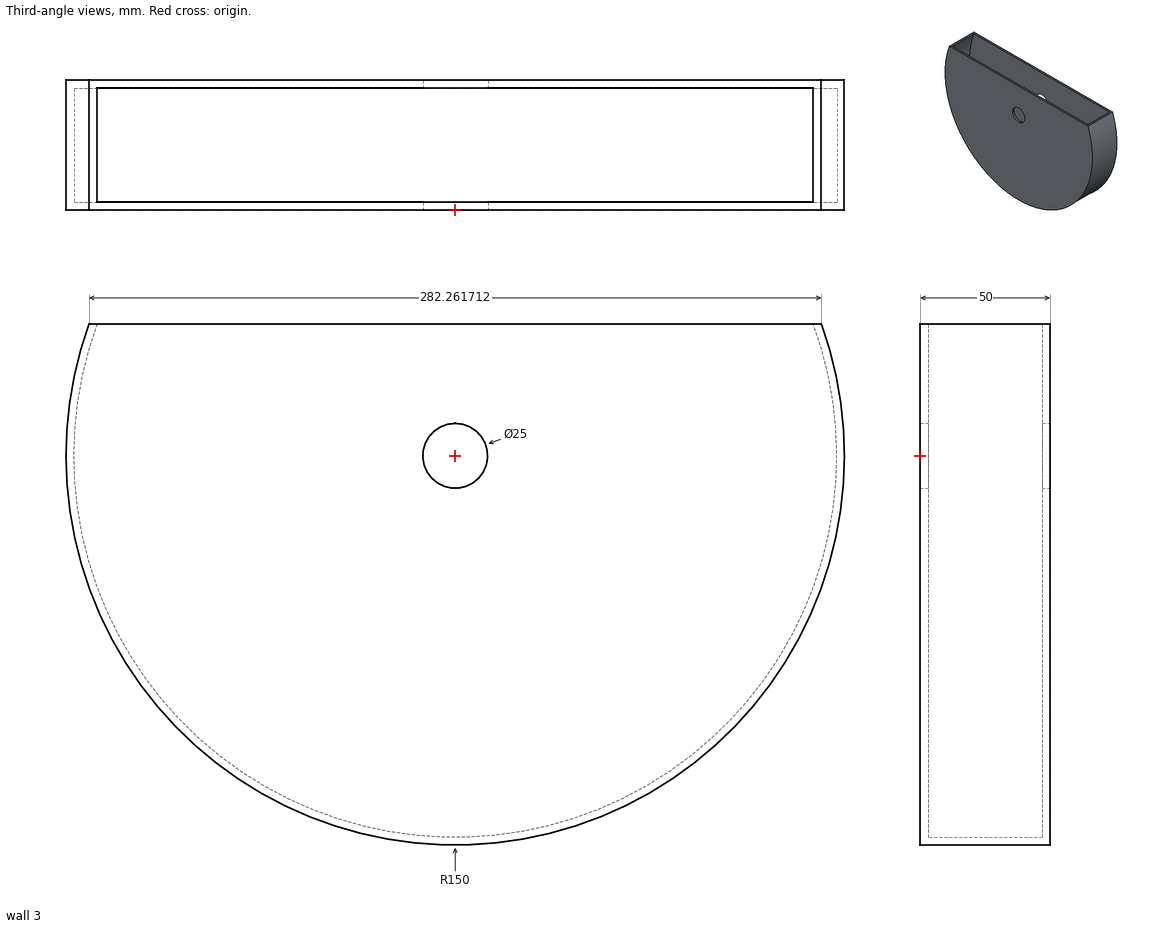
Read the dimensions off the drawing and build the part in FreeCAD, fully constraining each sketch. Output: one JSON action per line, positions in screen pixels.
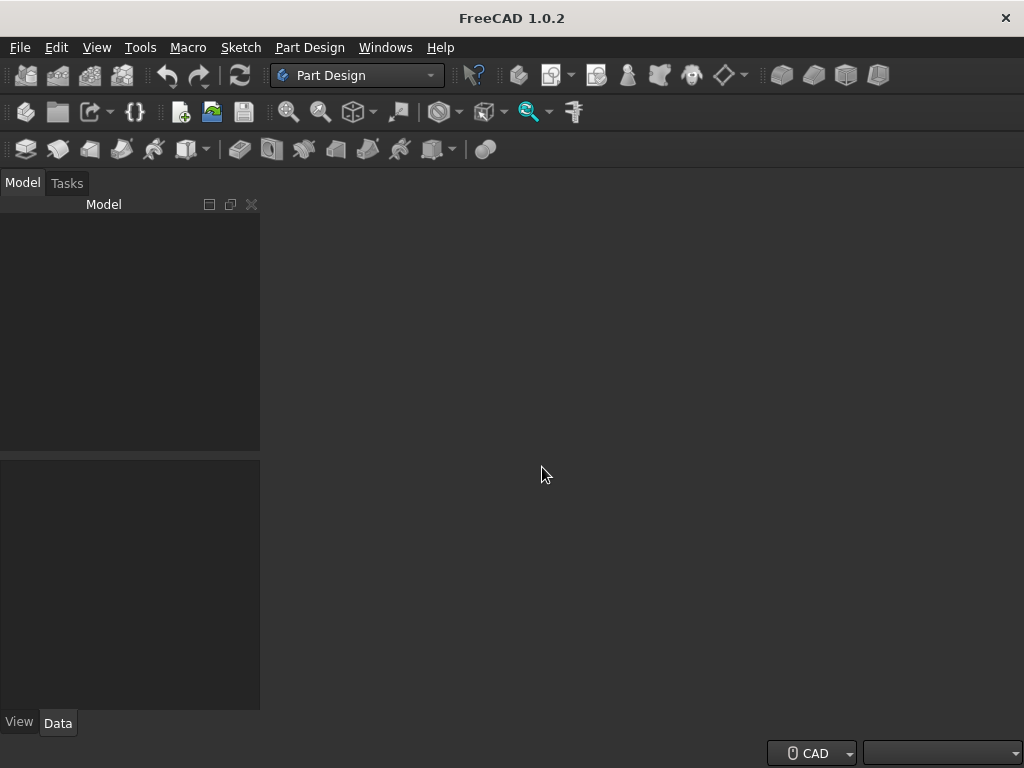
{"action": "key", "text": "ctrl+n"}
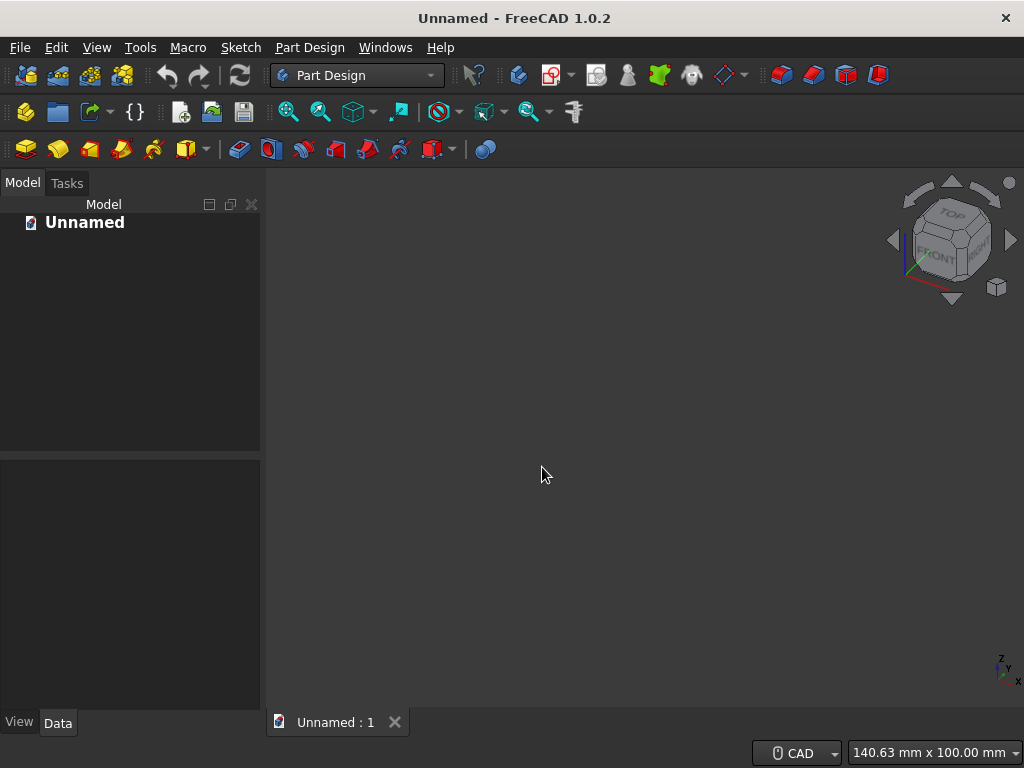
{"action": "left_click", "coordinate": [552, 76]}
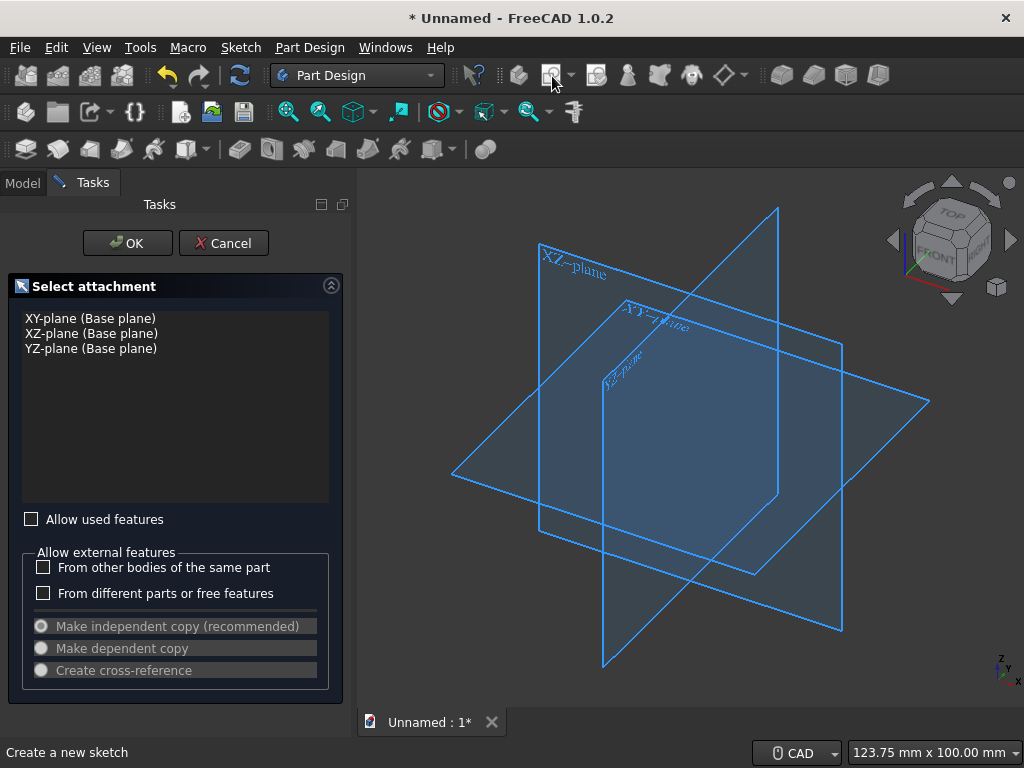
{"action": "left_click", "coordinate": [82, 334]}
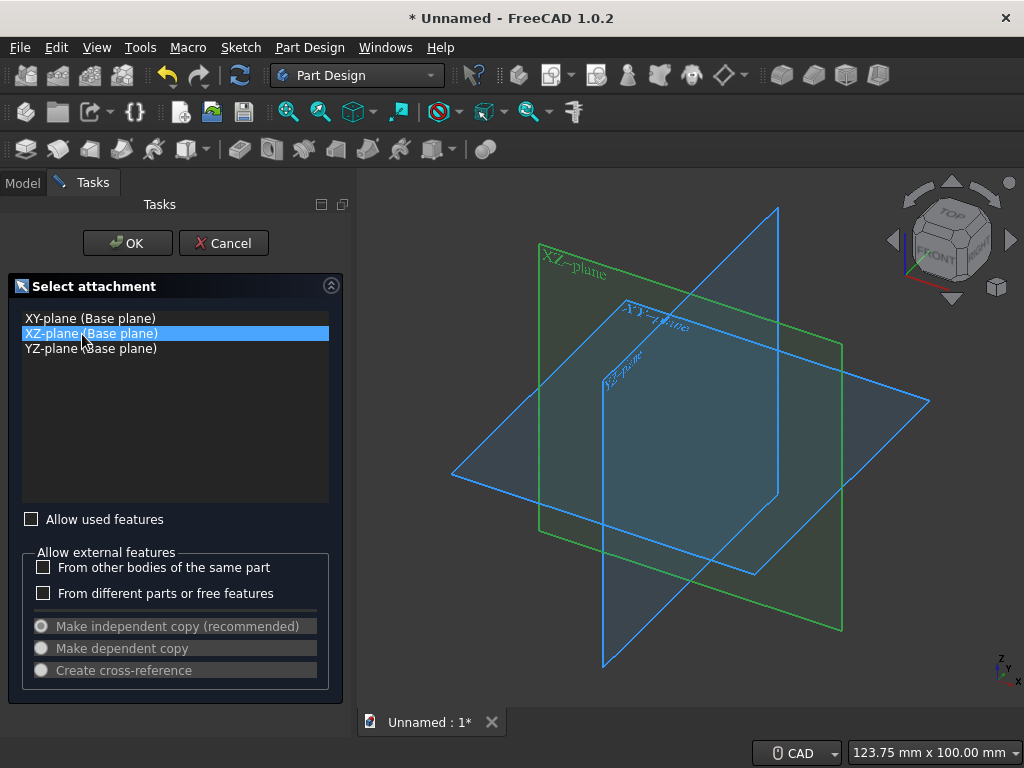
{"action": "left_click", "coordinate": [128, 243]}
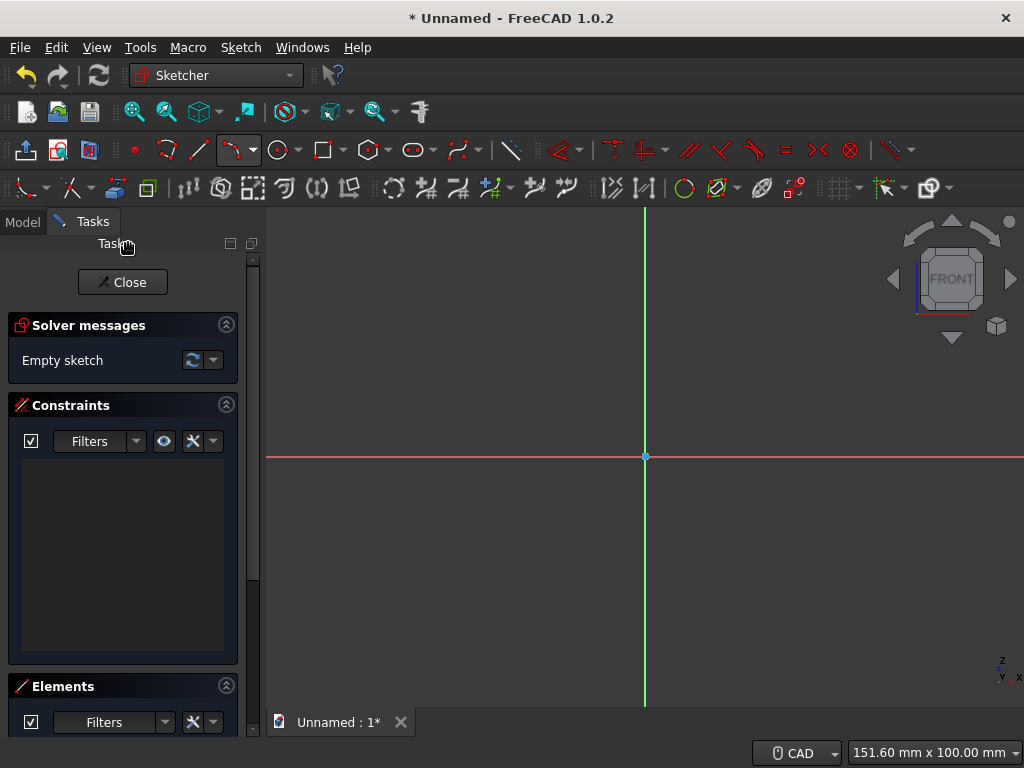
{"action": "scroll", "coordinate": [547, 350], "scroll_direction": "down", "scroll_amount": 6}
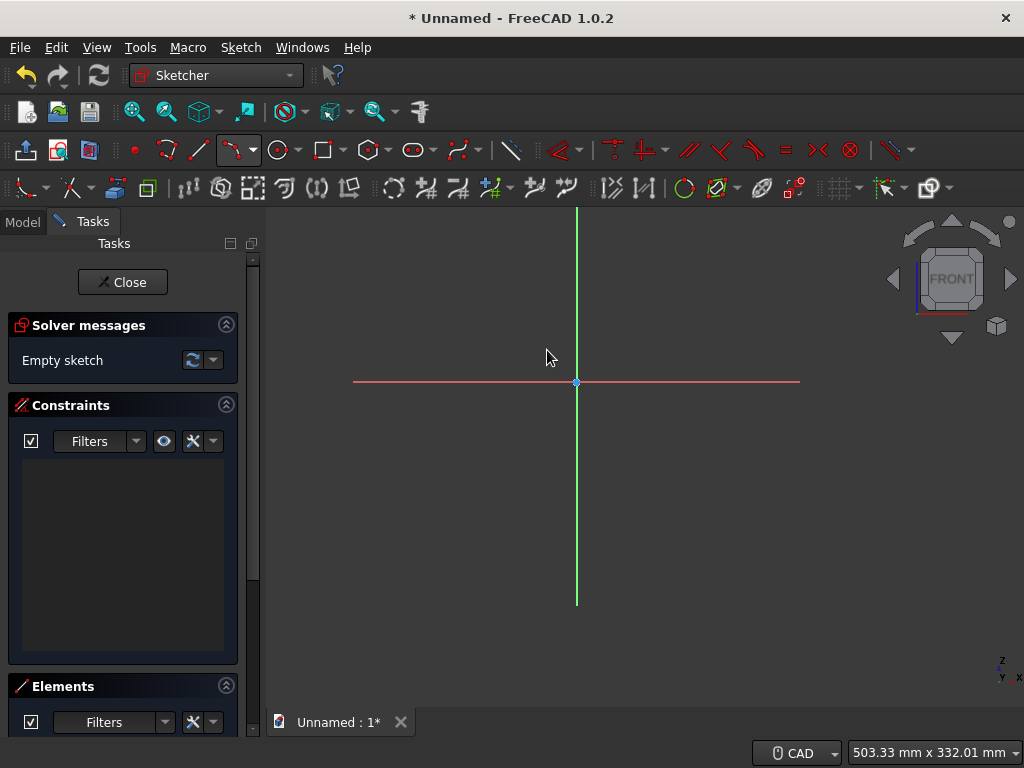
{"action": "left_click", "coordinate": [200, 150]}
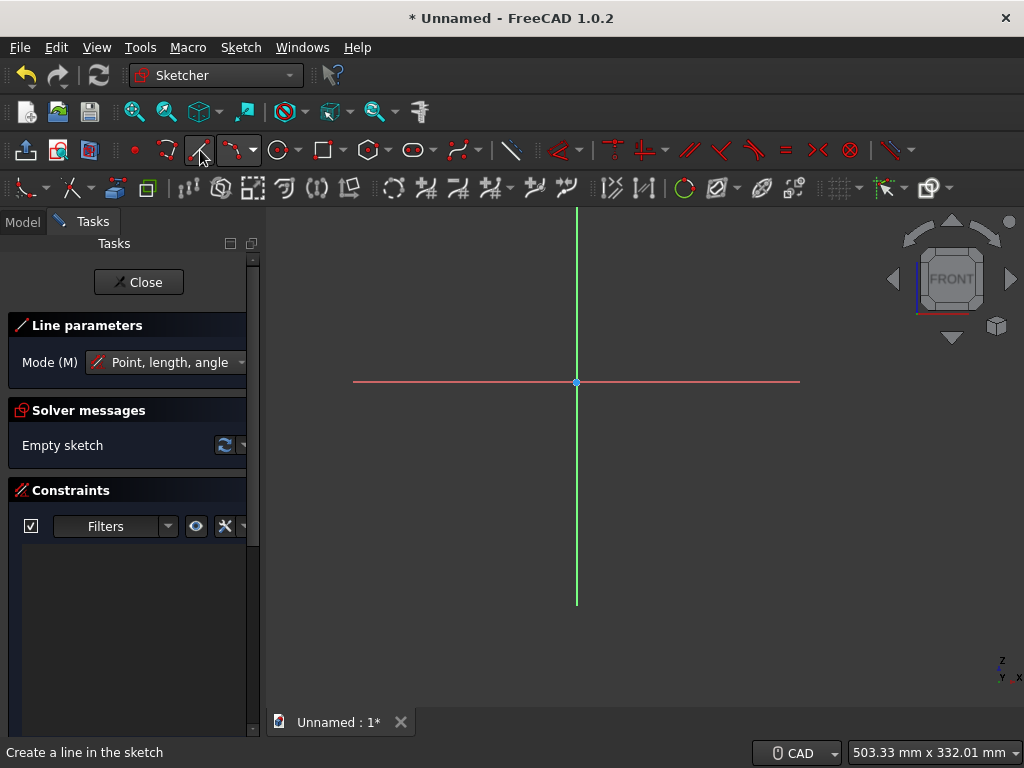
{"action": "left_click", "coordinate": [364, 306]}
{"action": "left_click", "coordinate": [789, 306]}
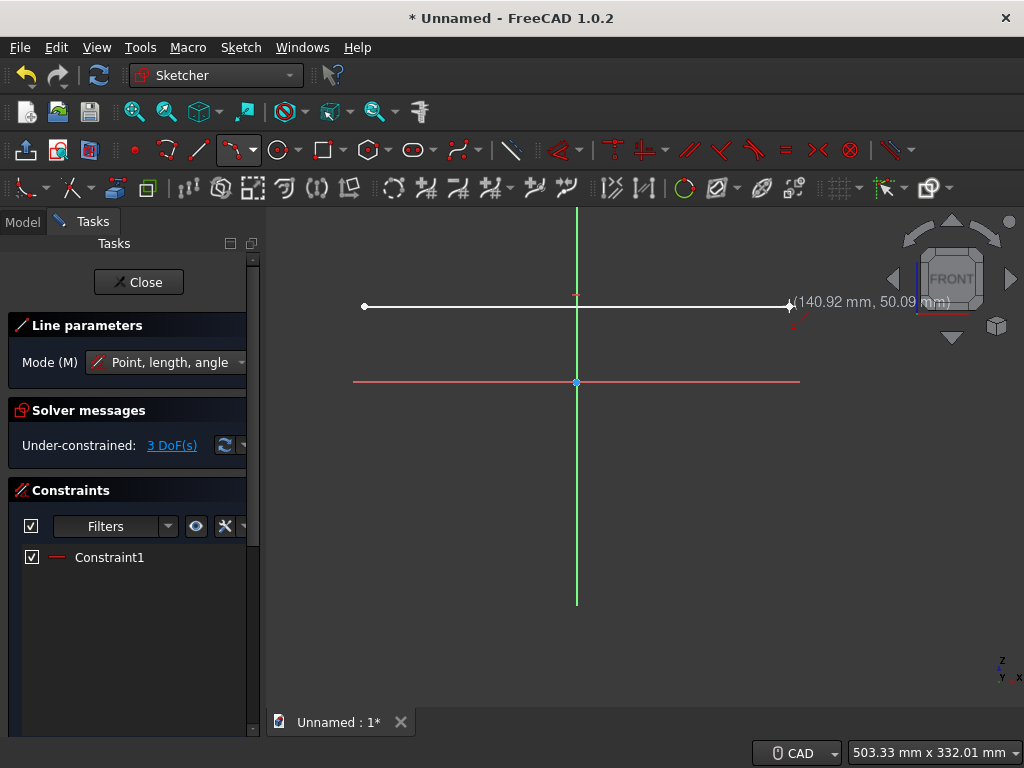
{"action": "key", "text": "g 3 a"}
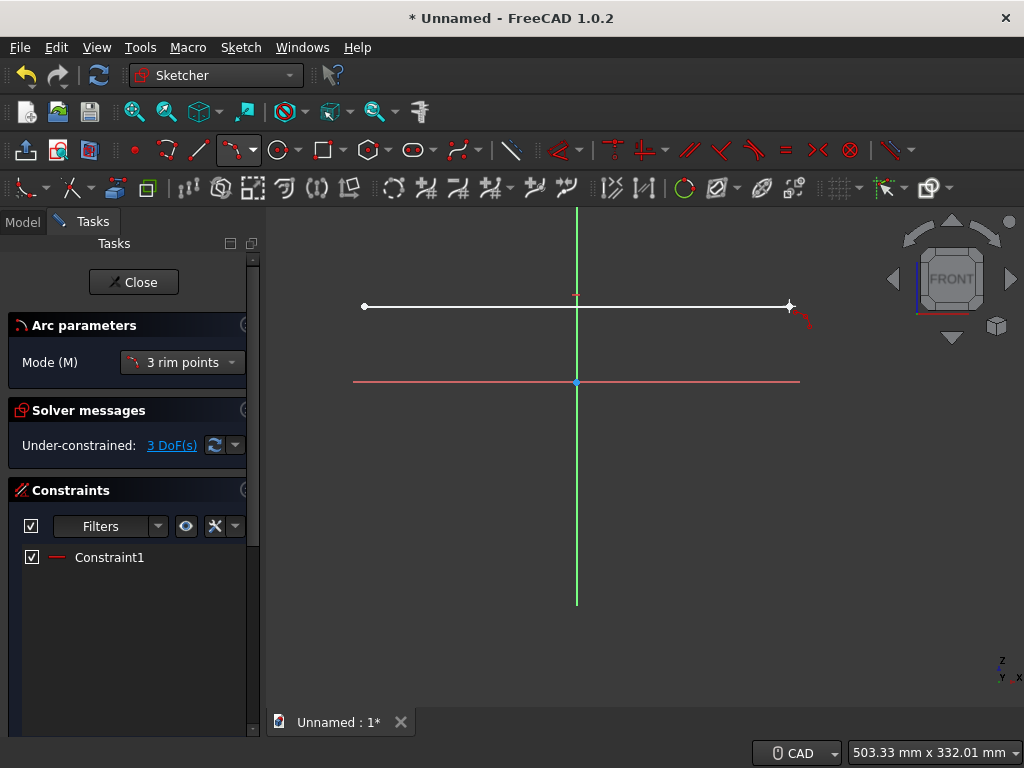
{"action": "left_click", "coordinate": [789, 307]}
{"action": "left_click", "coordinate": [364, 307]}
{"action": "left_click", "coordinate": [492, 592]}
{"action": "key", "text": "Escape"}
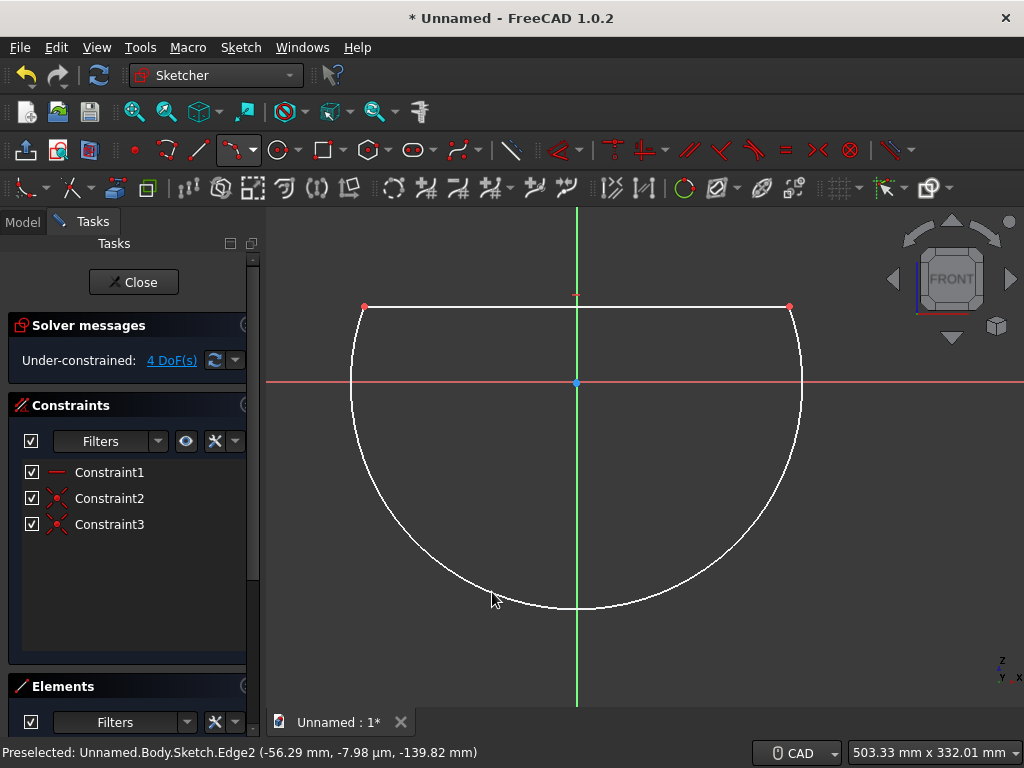
{"action": "left_click_drag", "start_coordinate": [566, 372], "coordinate": [587, 394]}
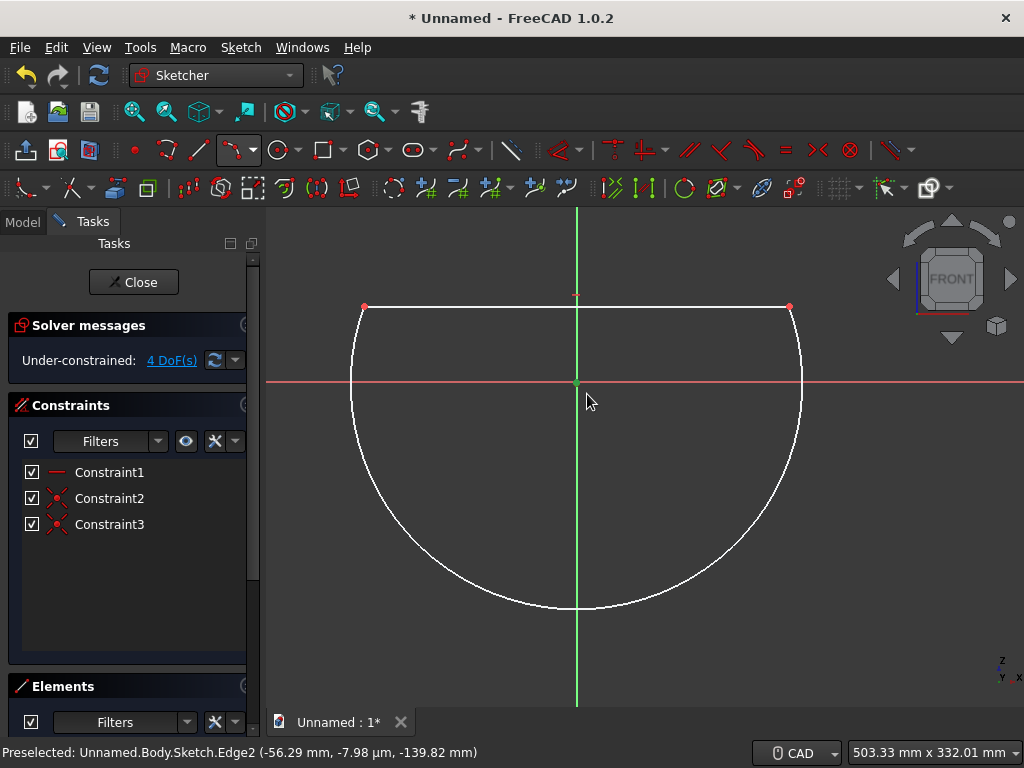
{"action": "key", "text": "c"}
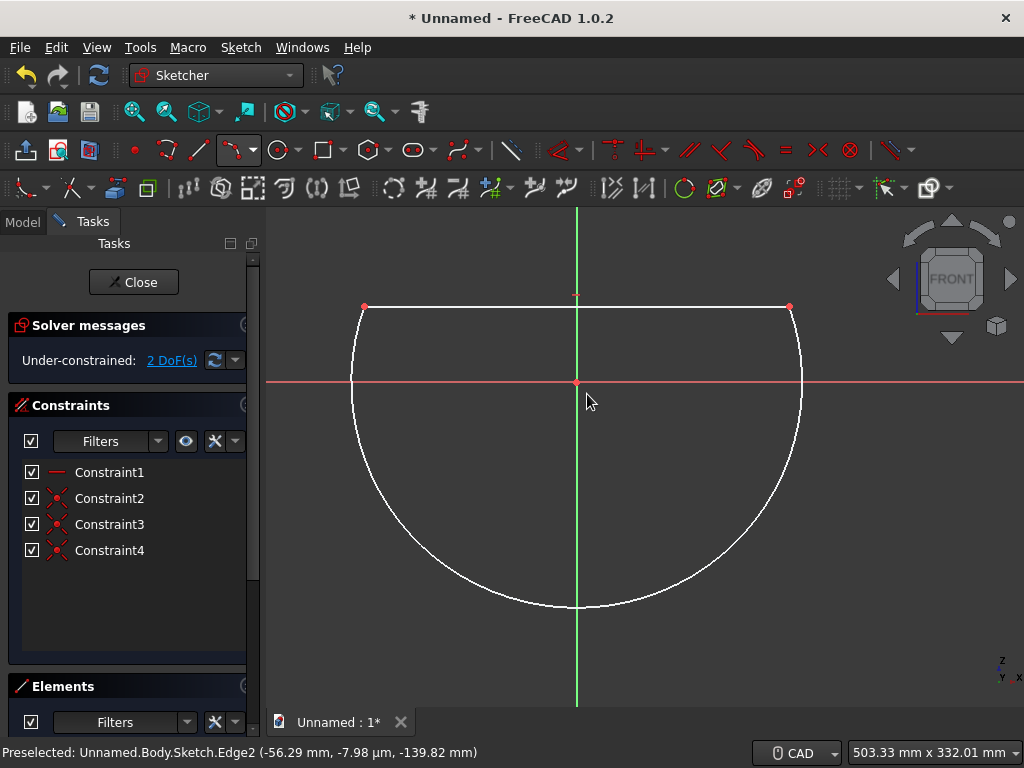
{"action": "left_click", "coordinate": [558, 150]}